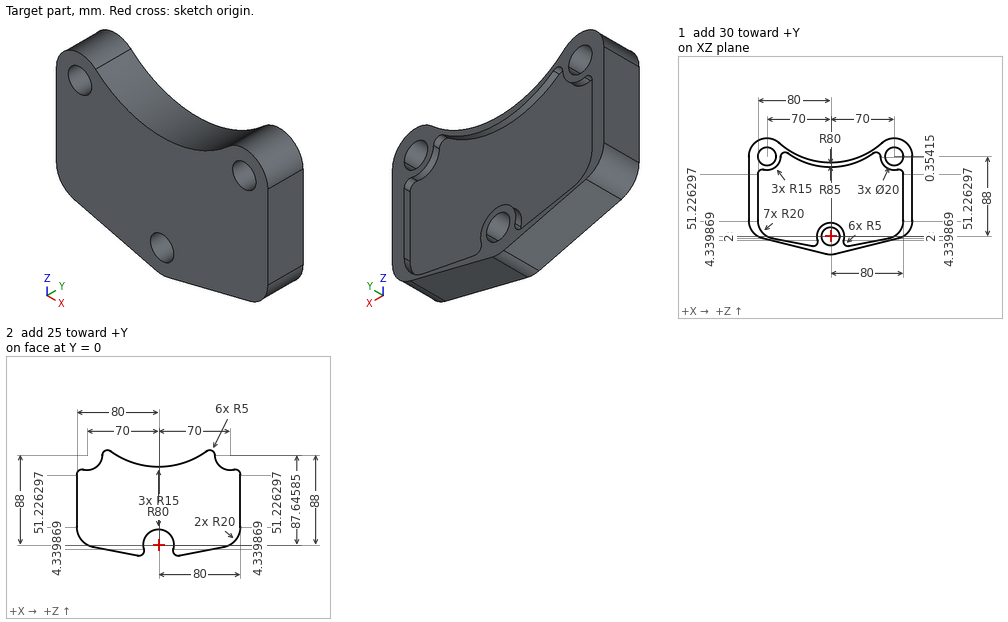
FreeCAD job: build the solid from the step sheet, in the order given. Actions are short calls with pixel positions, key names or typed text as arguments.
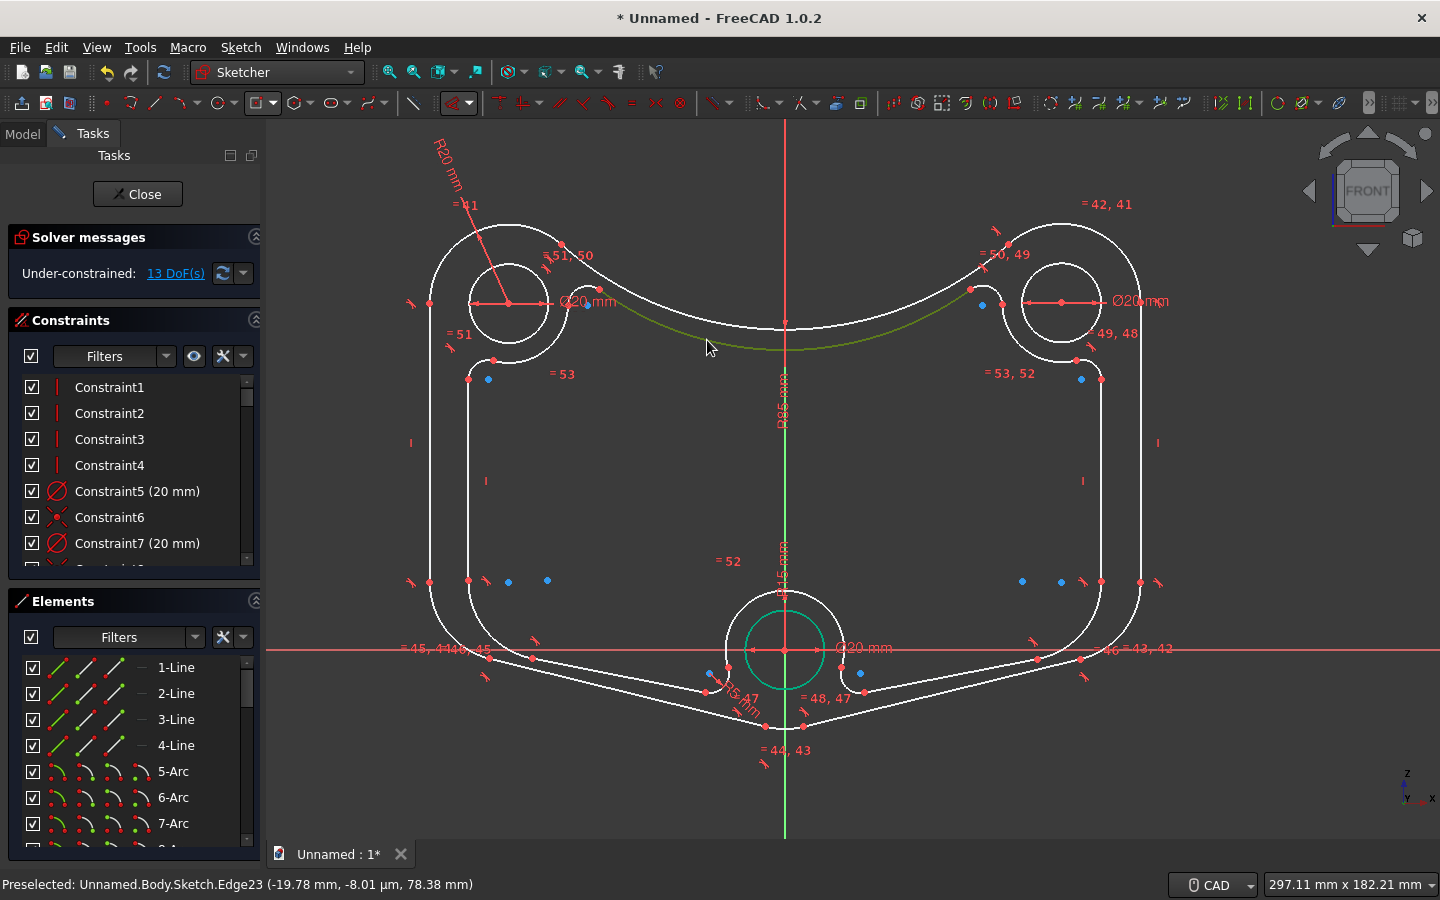
click(472, 104)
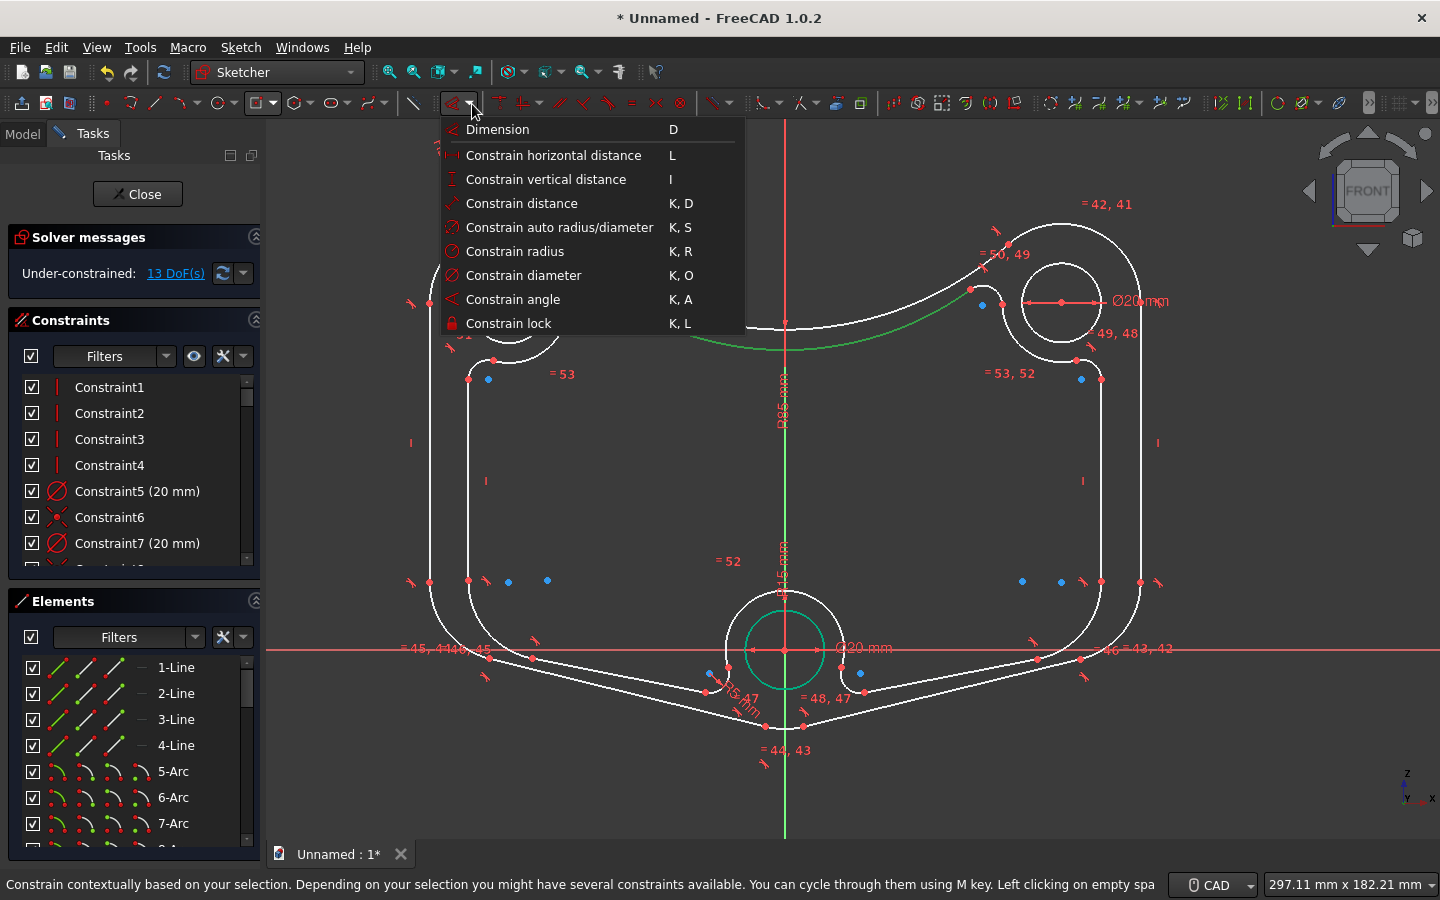
click(593, 251)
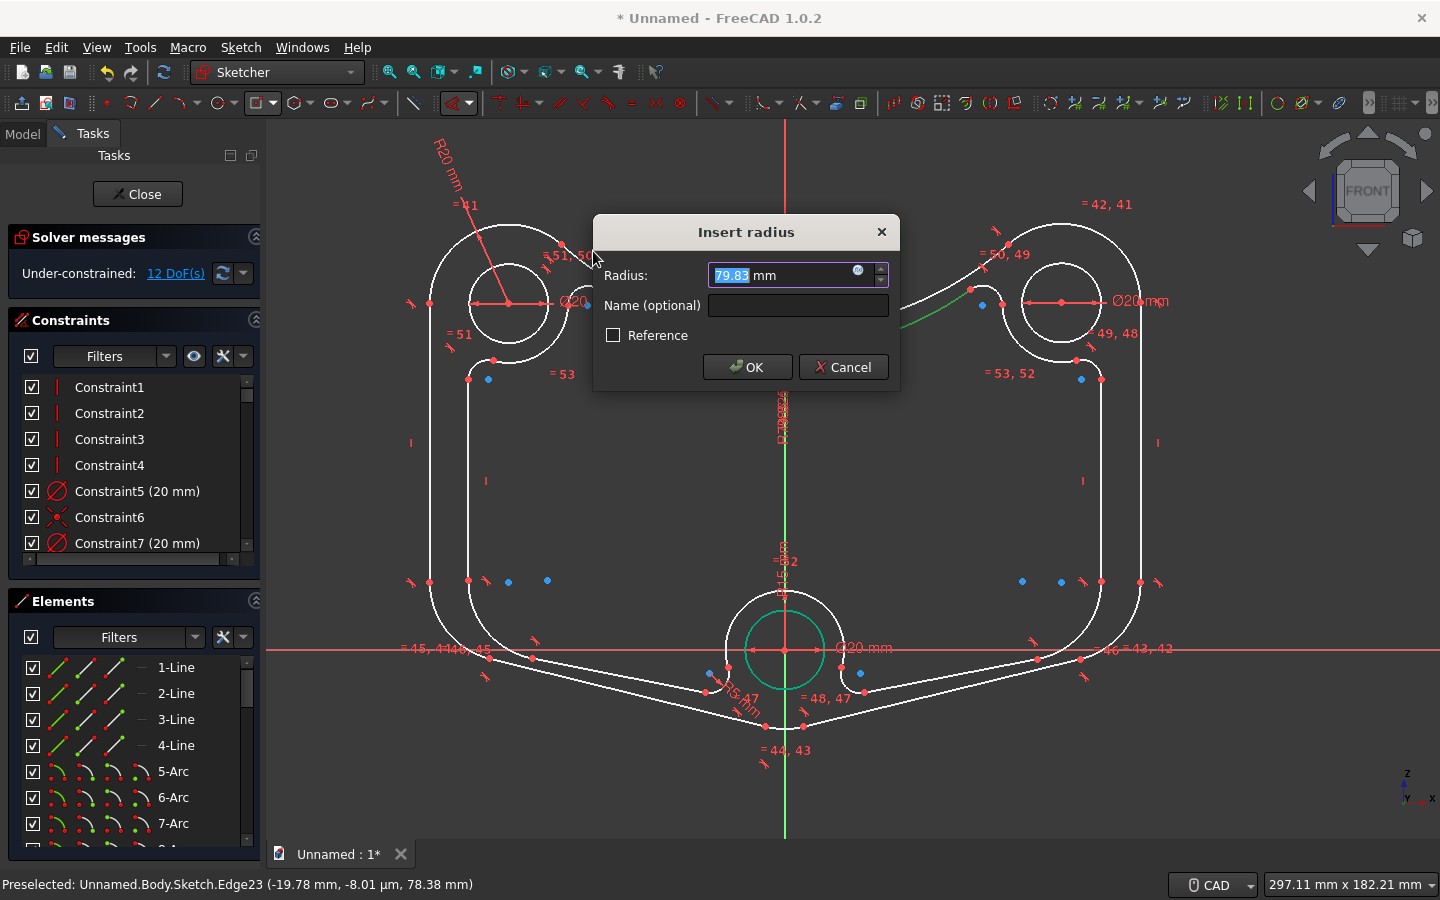
text(80)
key(Return)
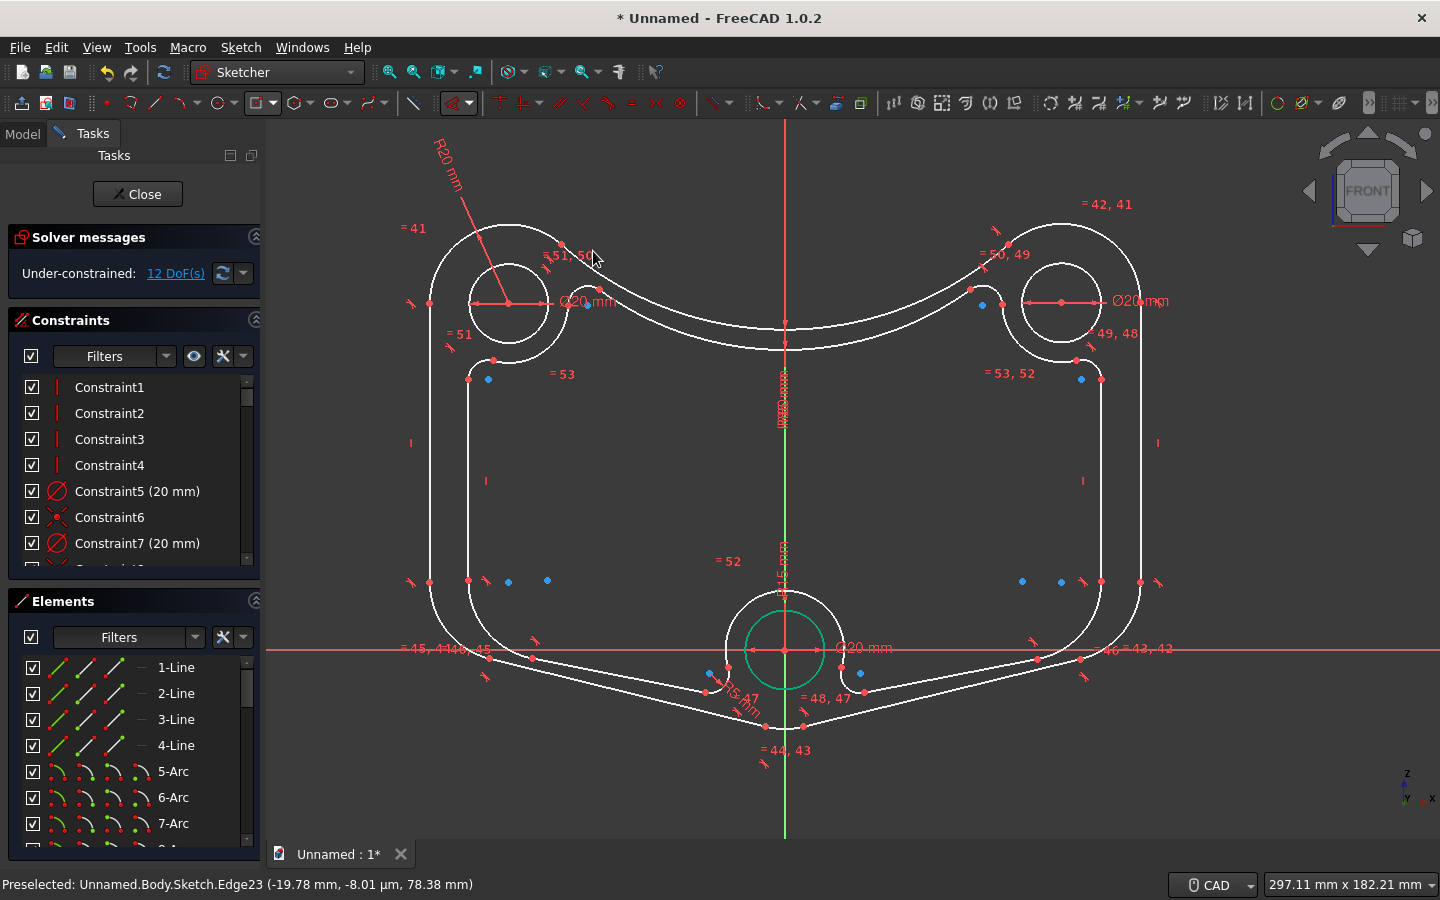
scroll(1080, 659, up, 9)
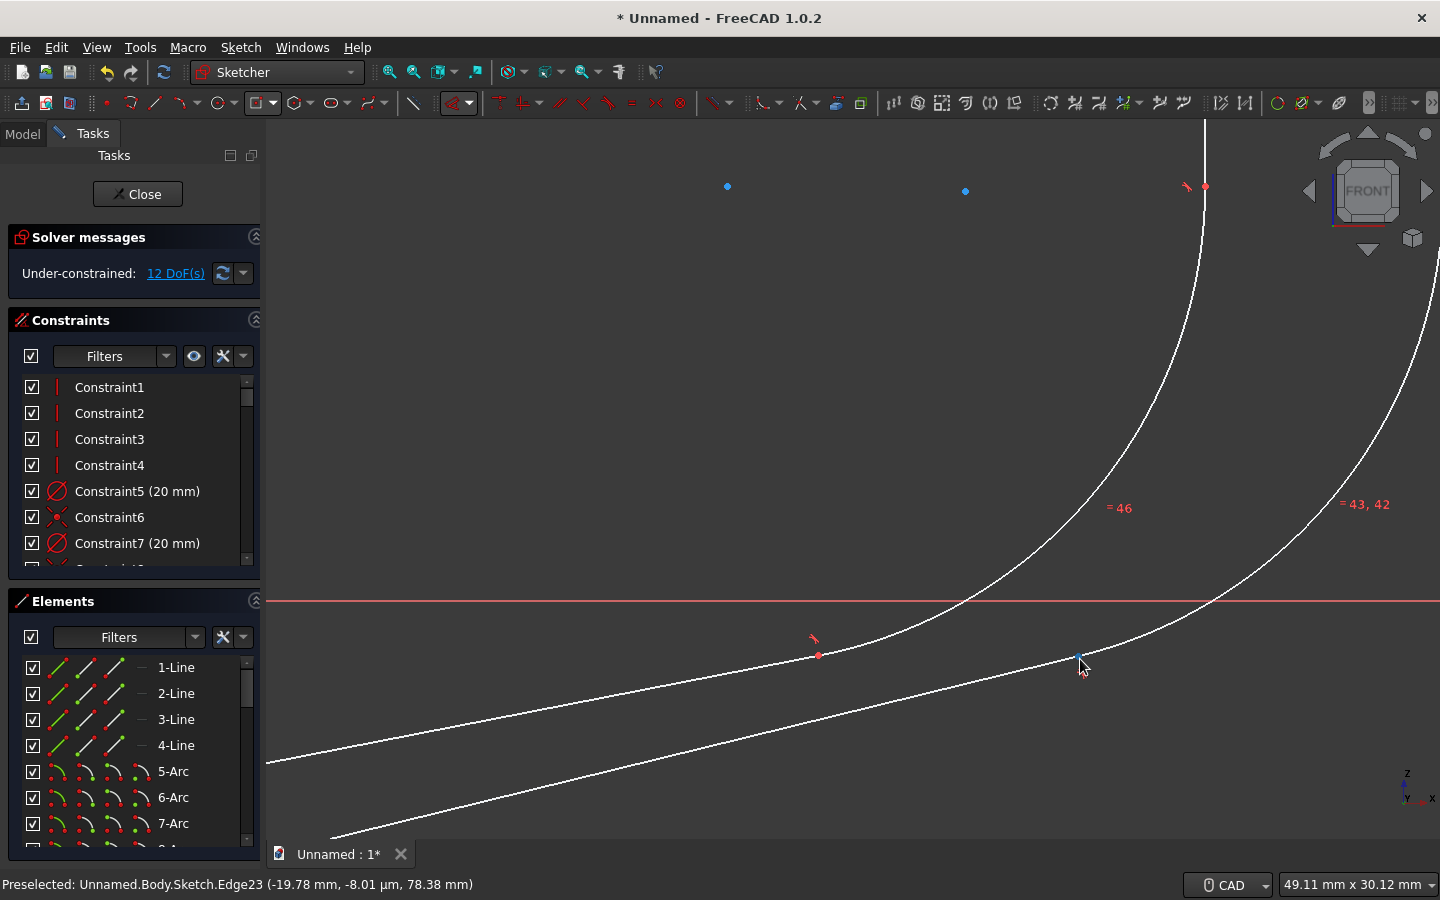
click(1079, 656)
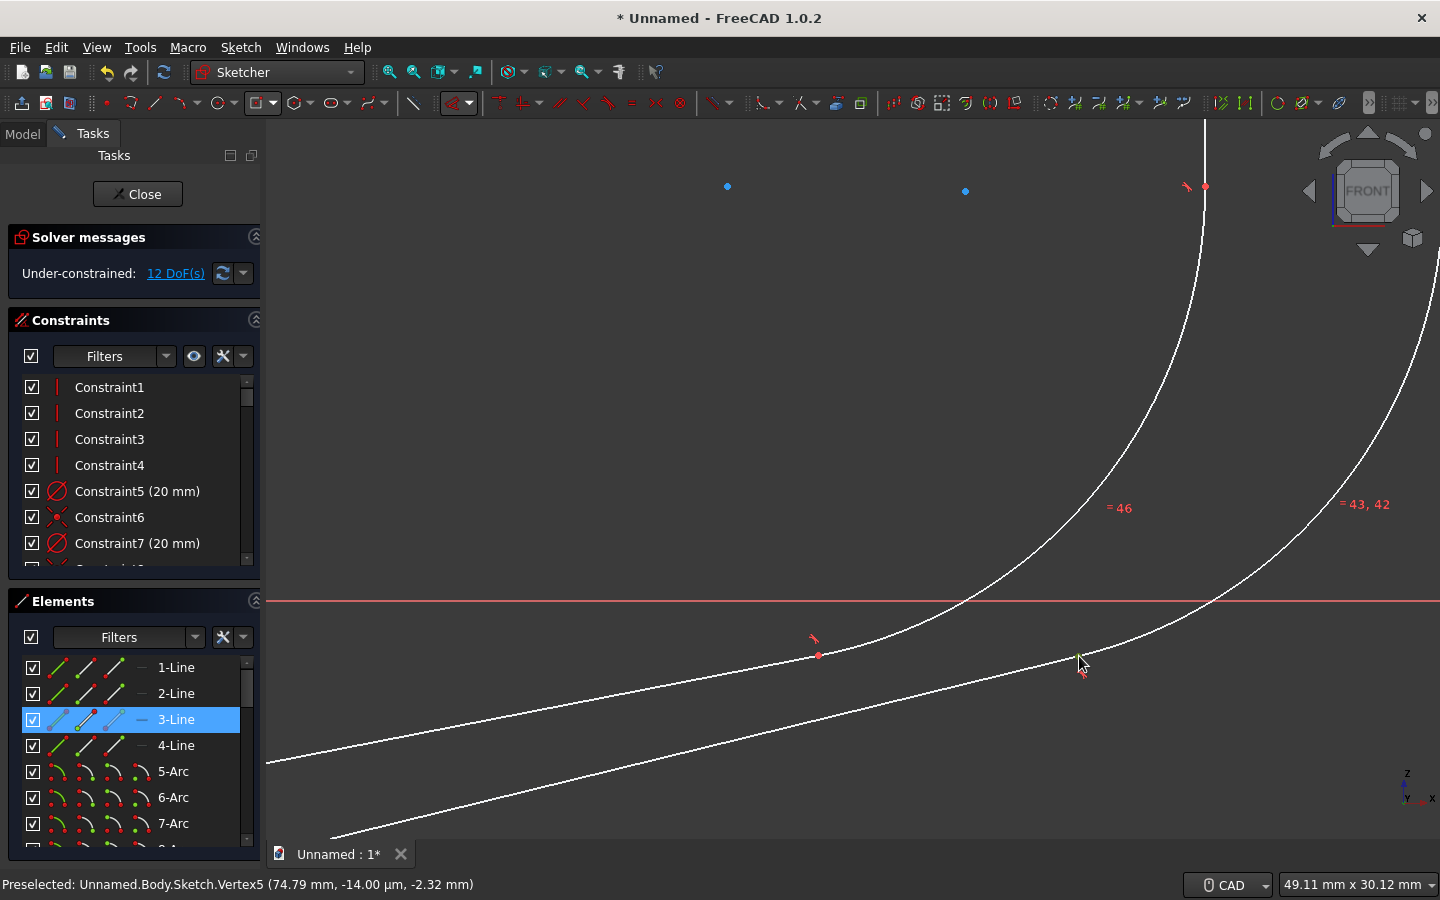
key(i)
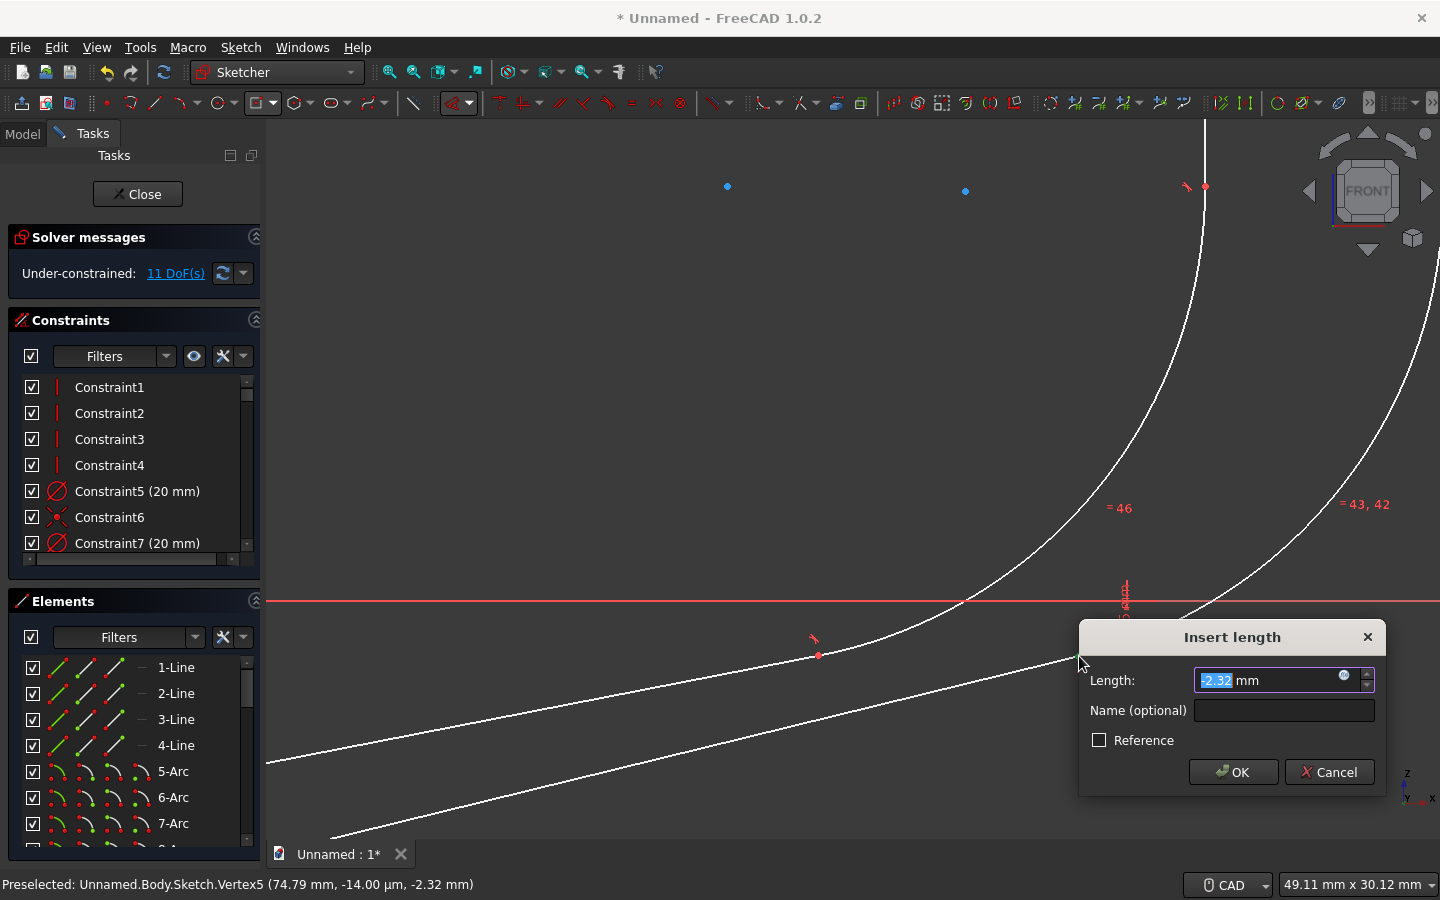
text(-2)
key(Return)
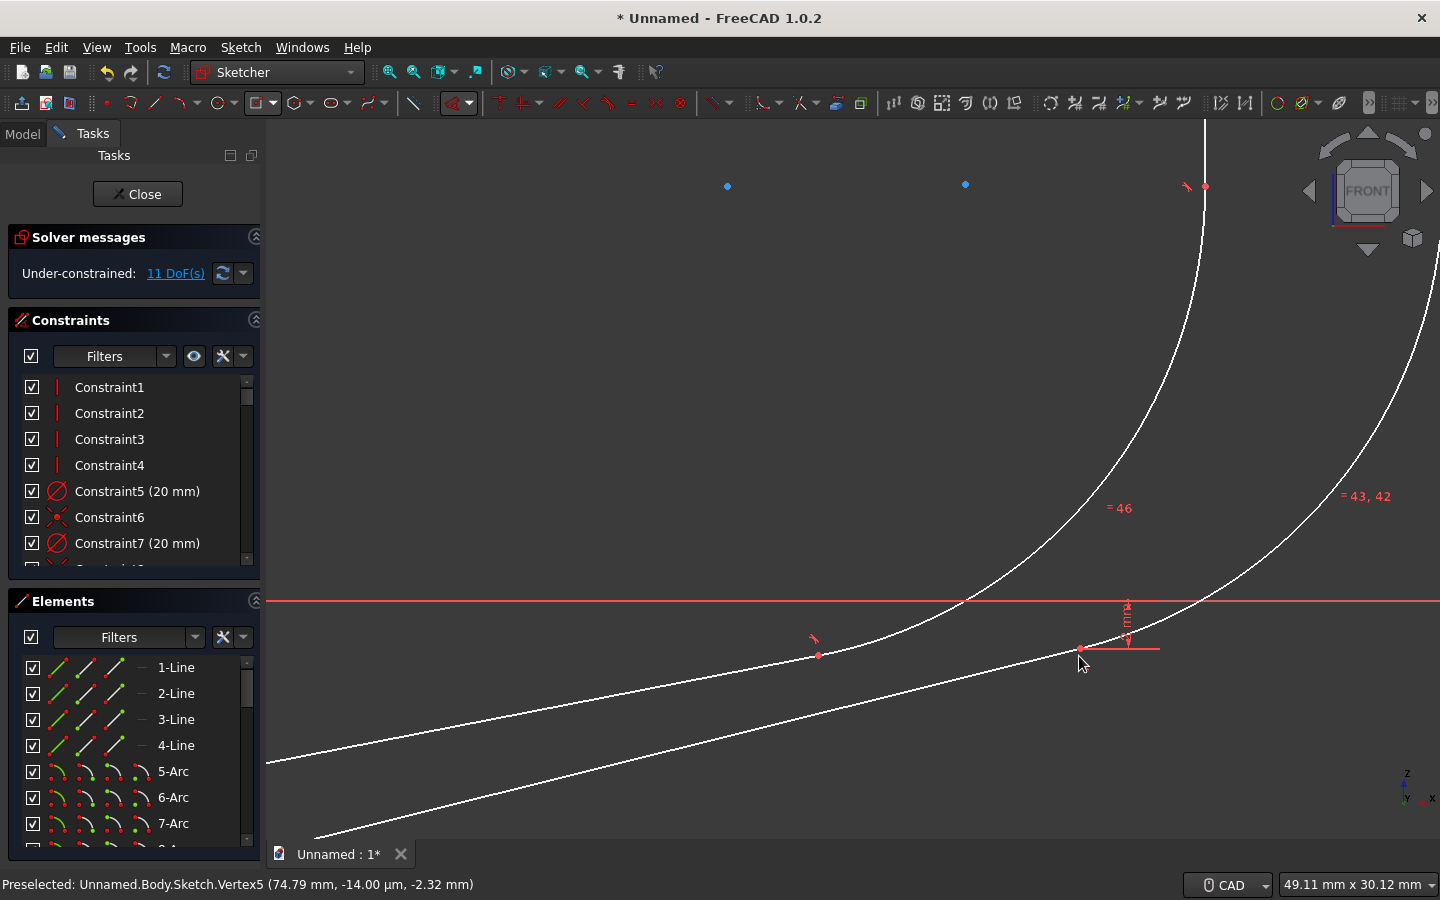
scroll(1080, 659, down, 9)